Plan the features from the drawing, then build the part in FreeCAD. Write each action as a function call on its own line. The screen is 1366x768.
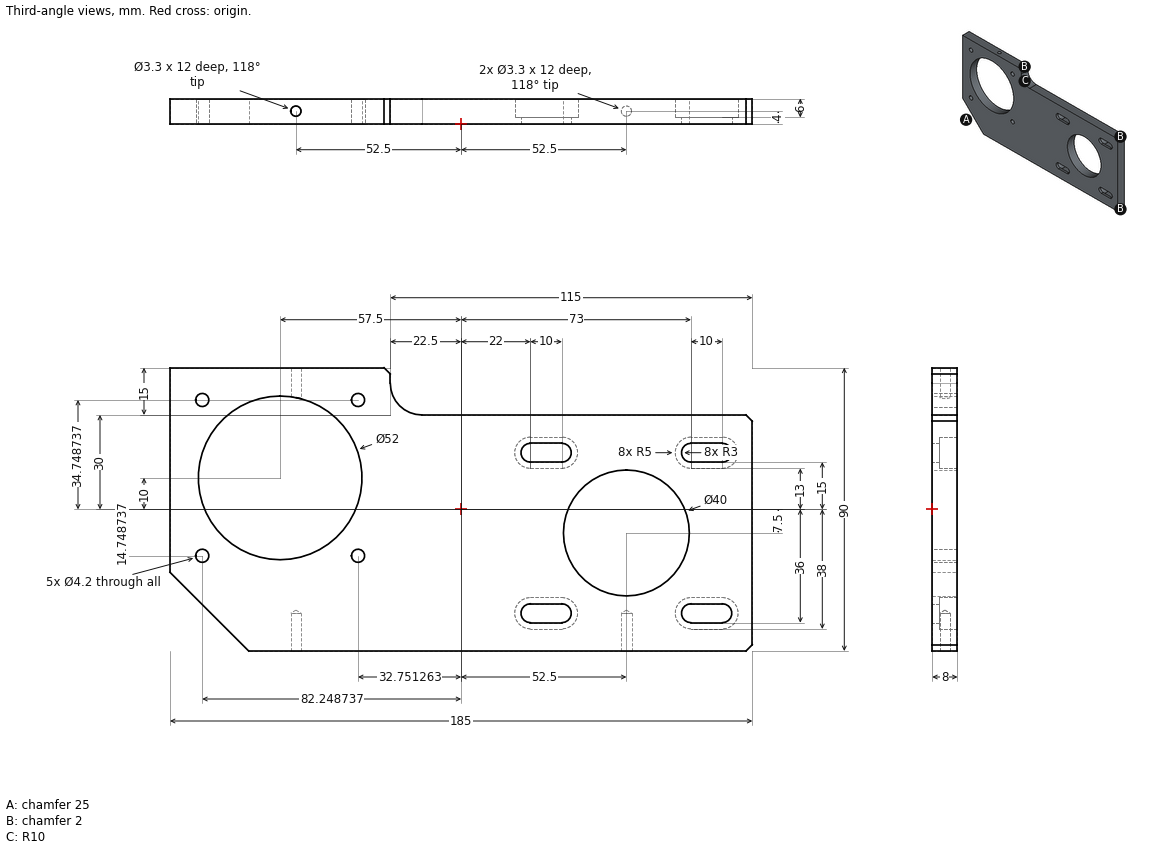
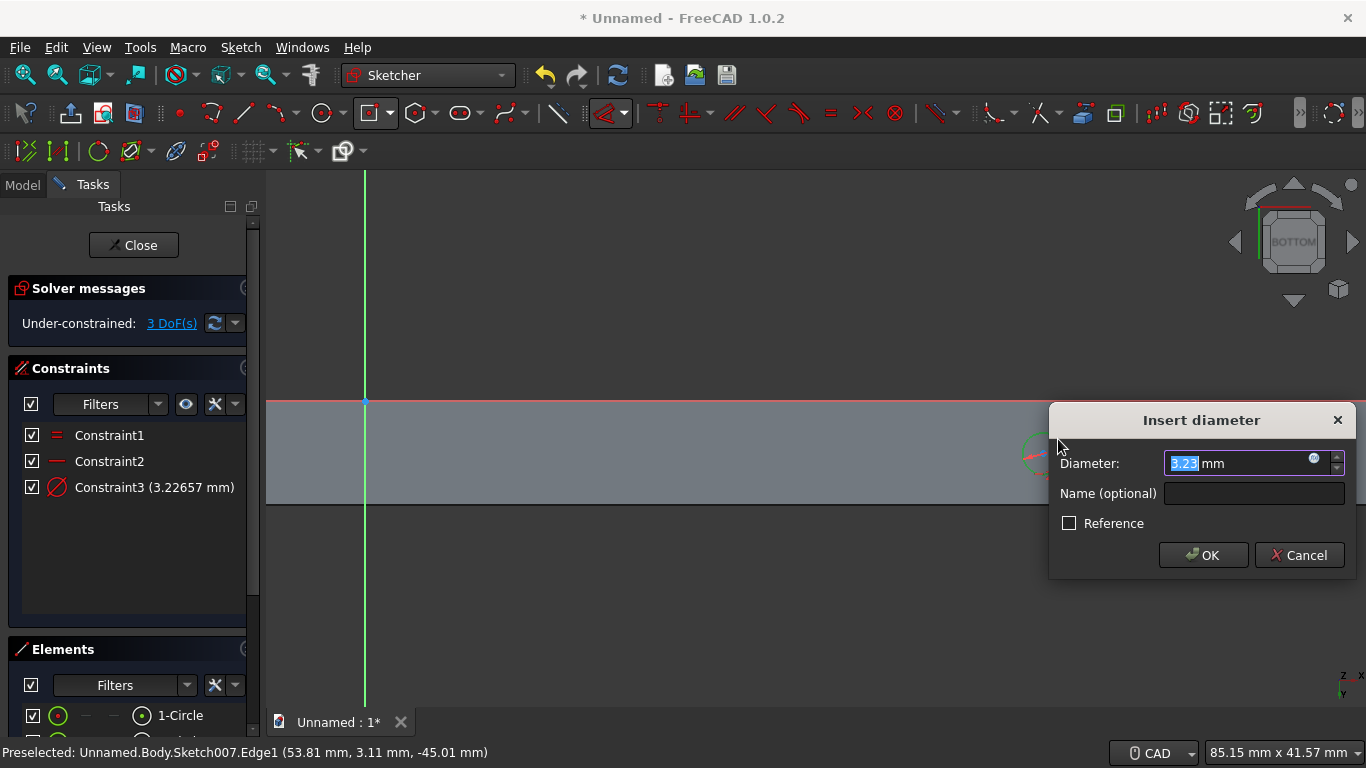
text(3.3)
key(Return)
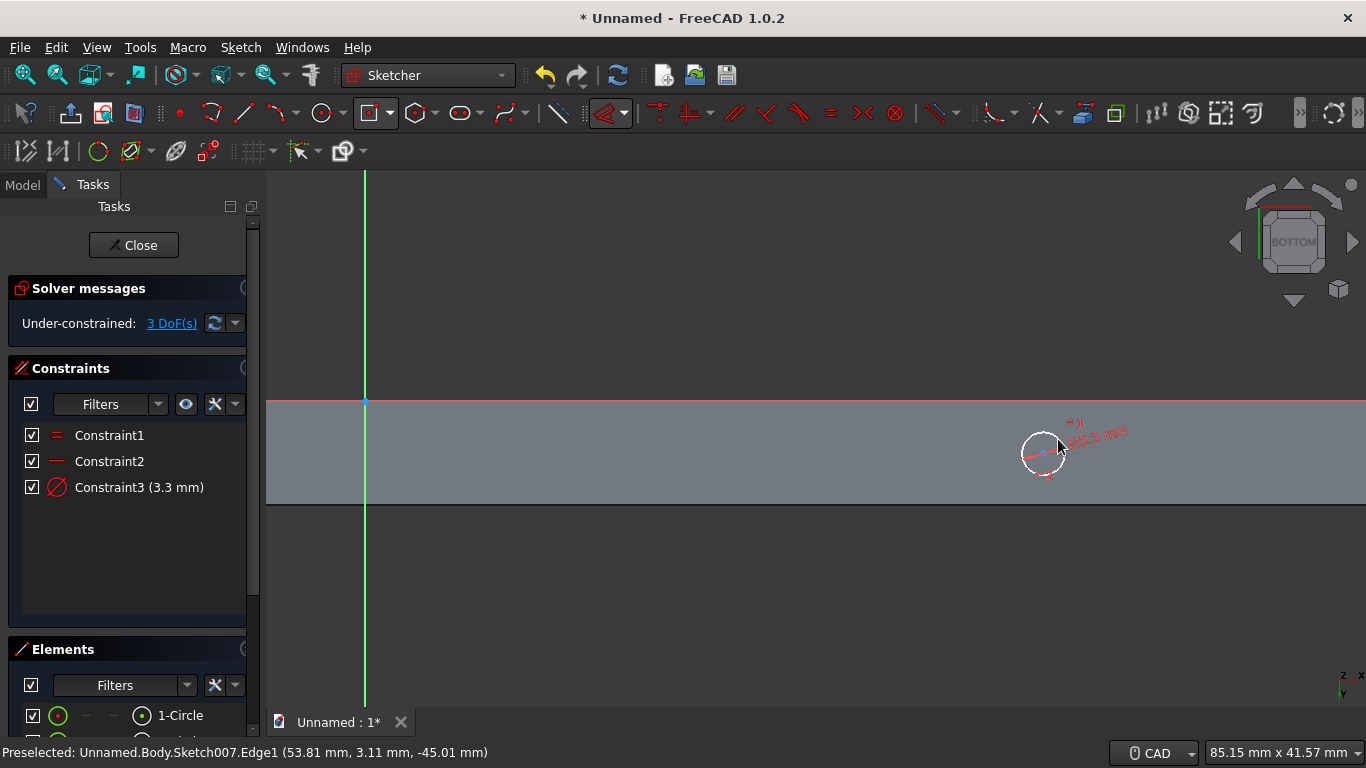
click(1043, 454)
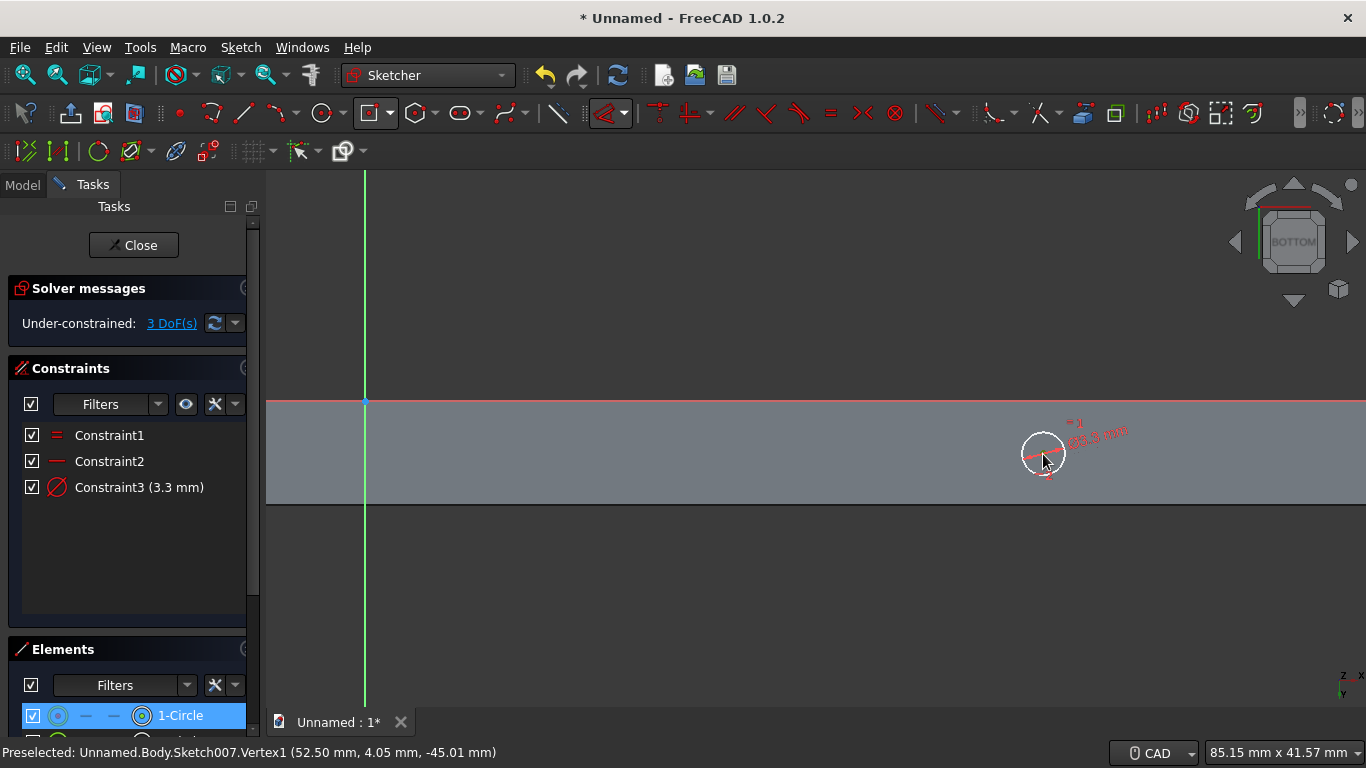
key(i)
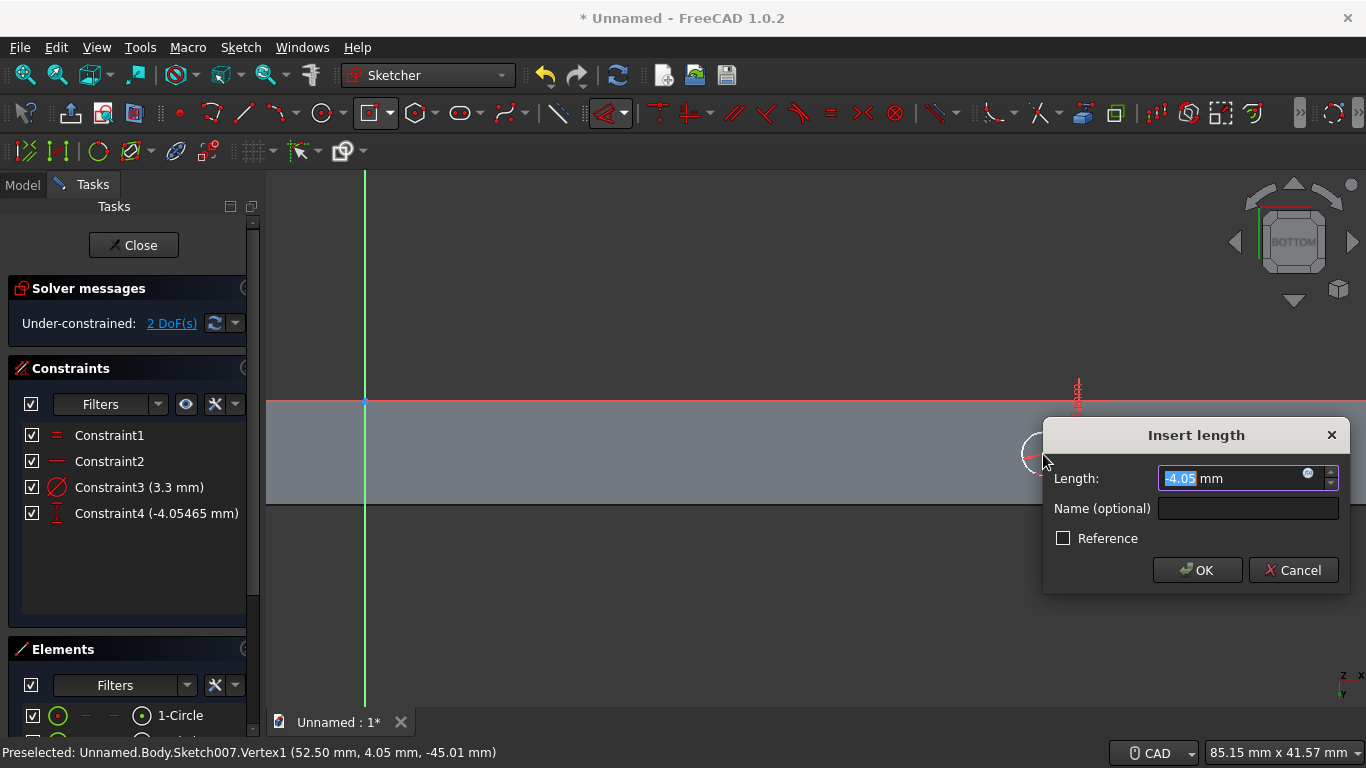
text(-4)
key(Return)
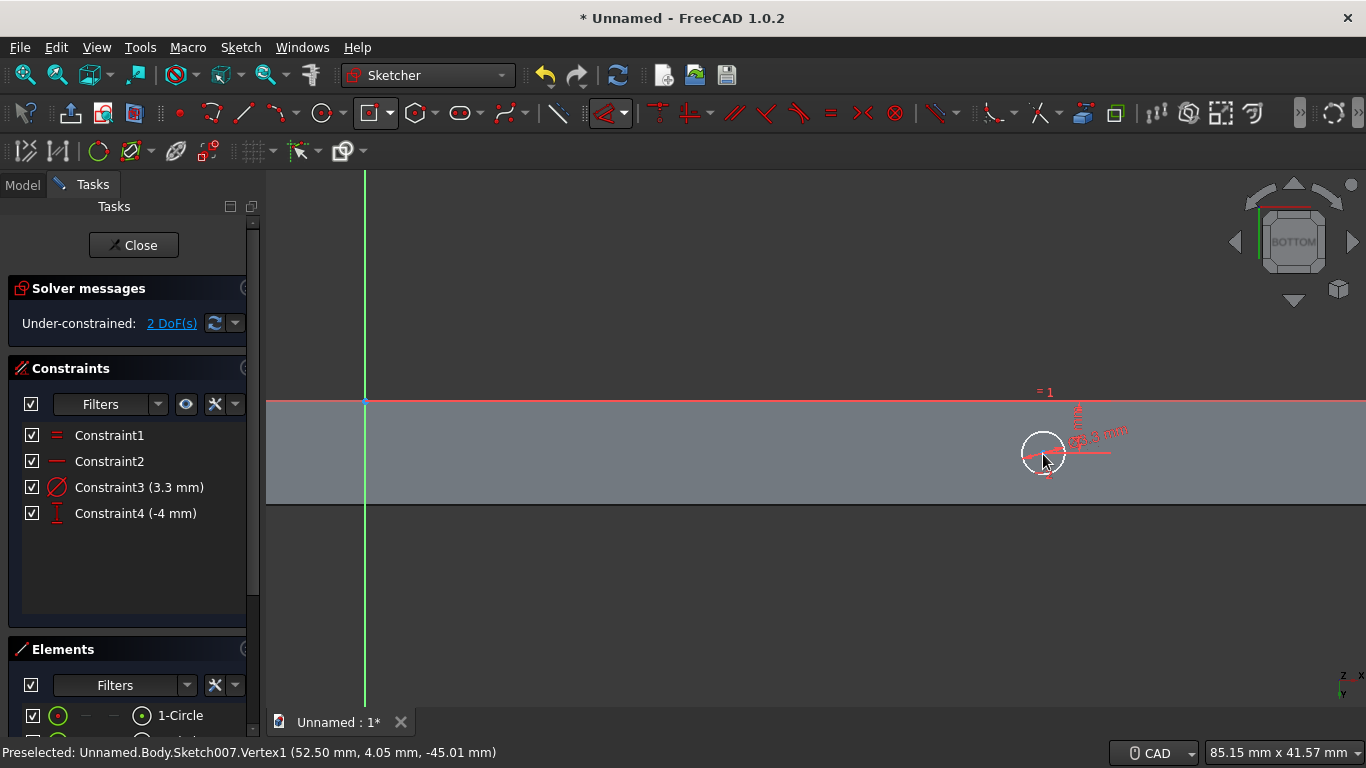
click(1043, 453)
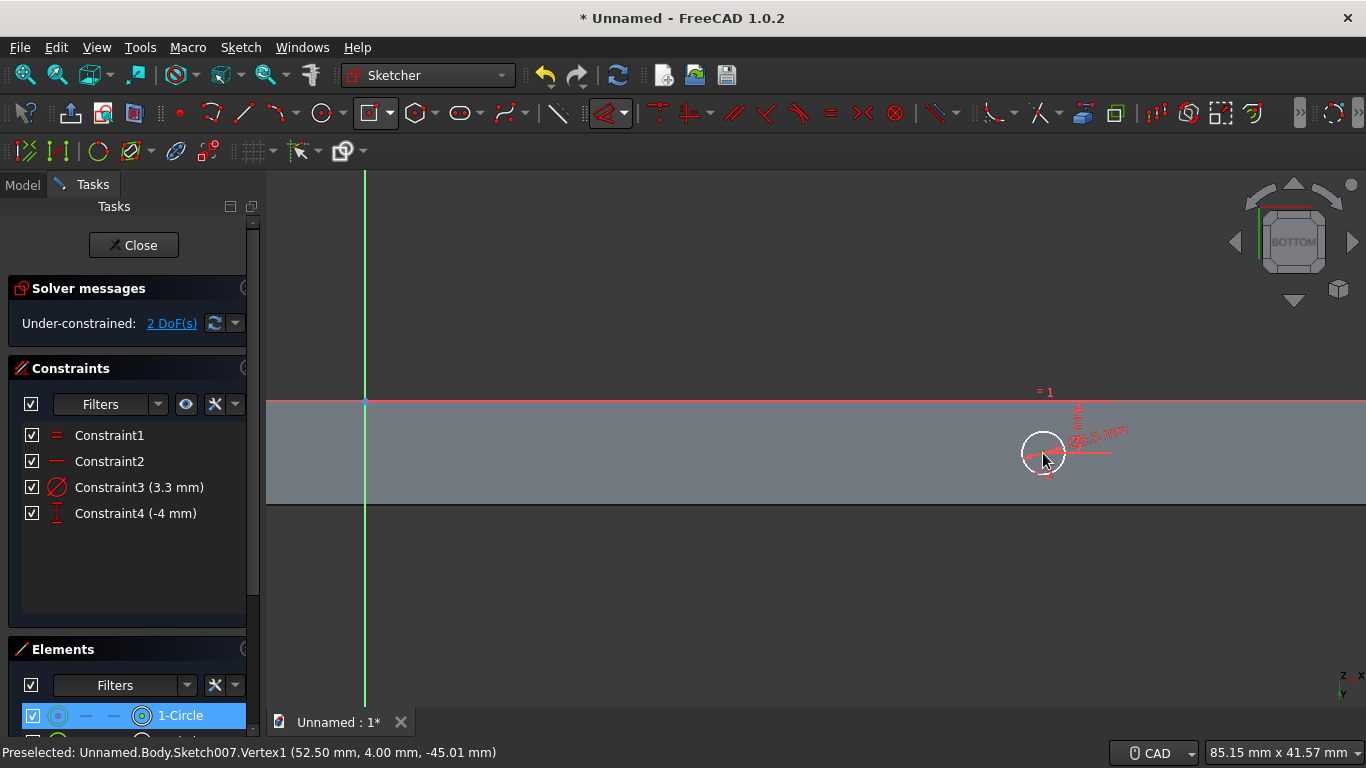
click(626, 114)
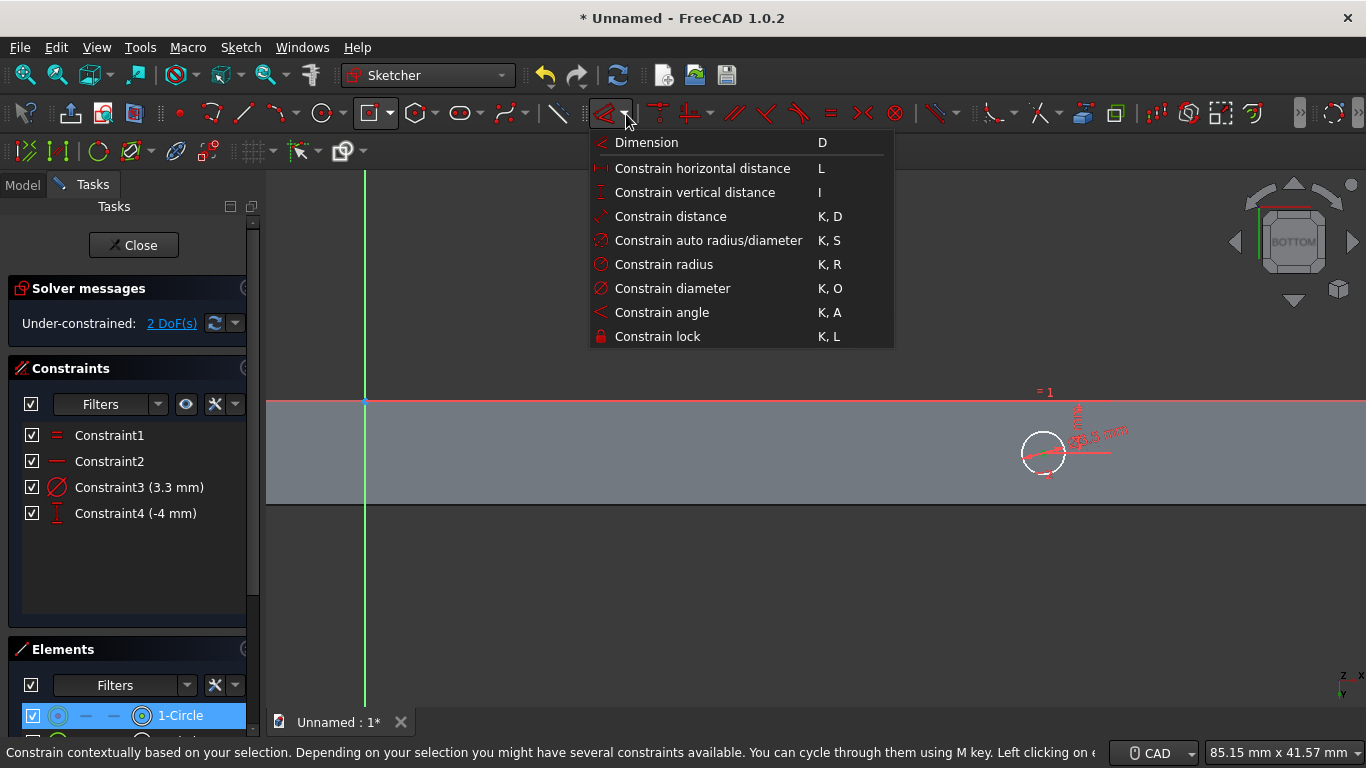
click(742, 168)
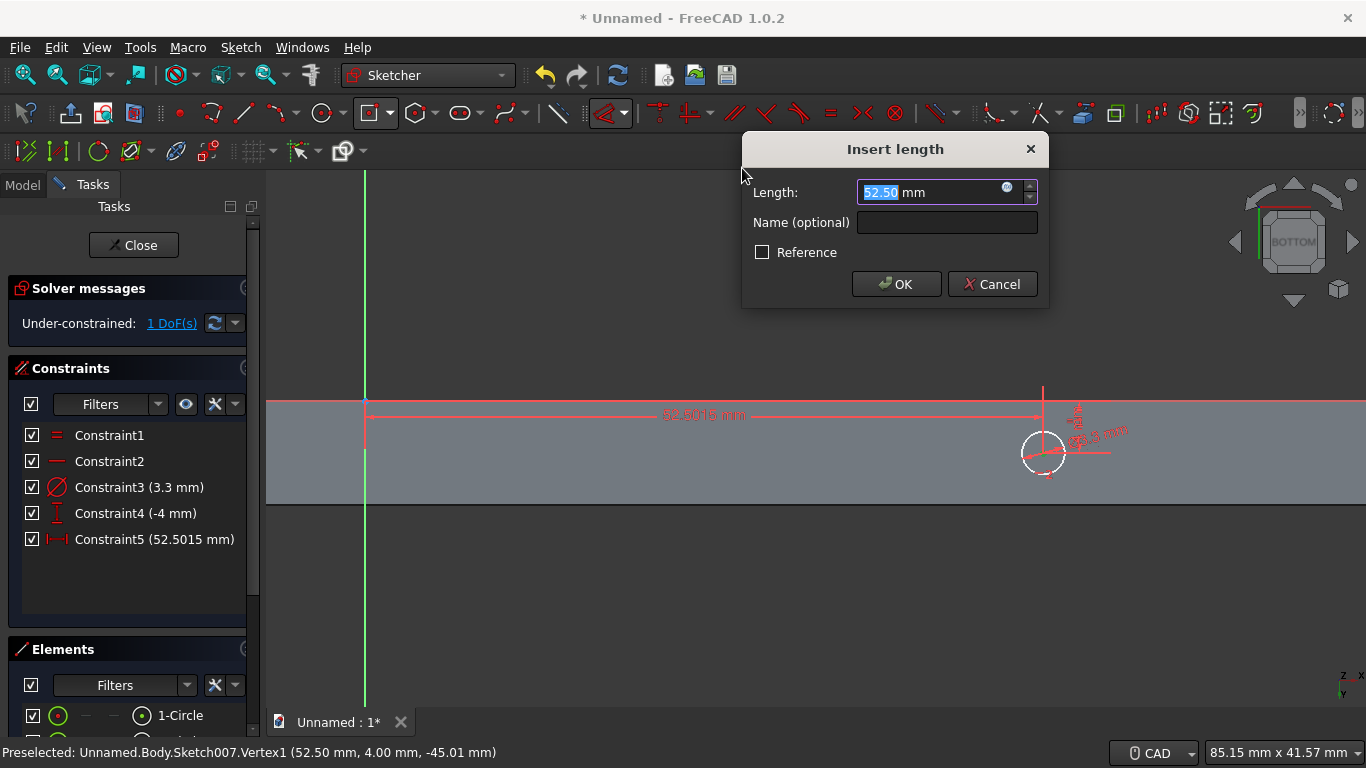
text(52.5)
key(Return)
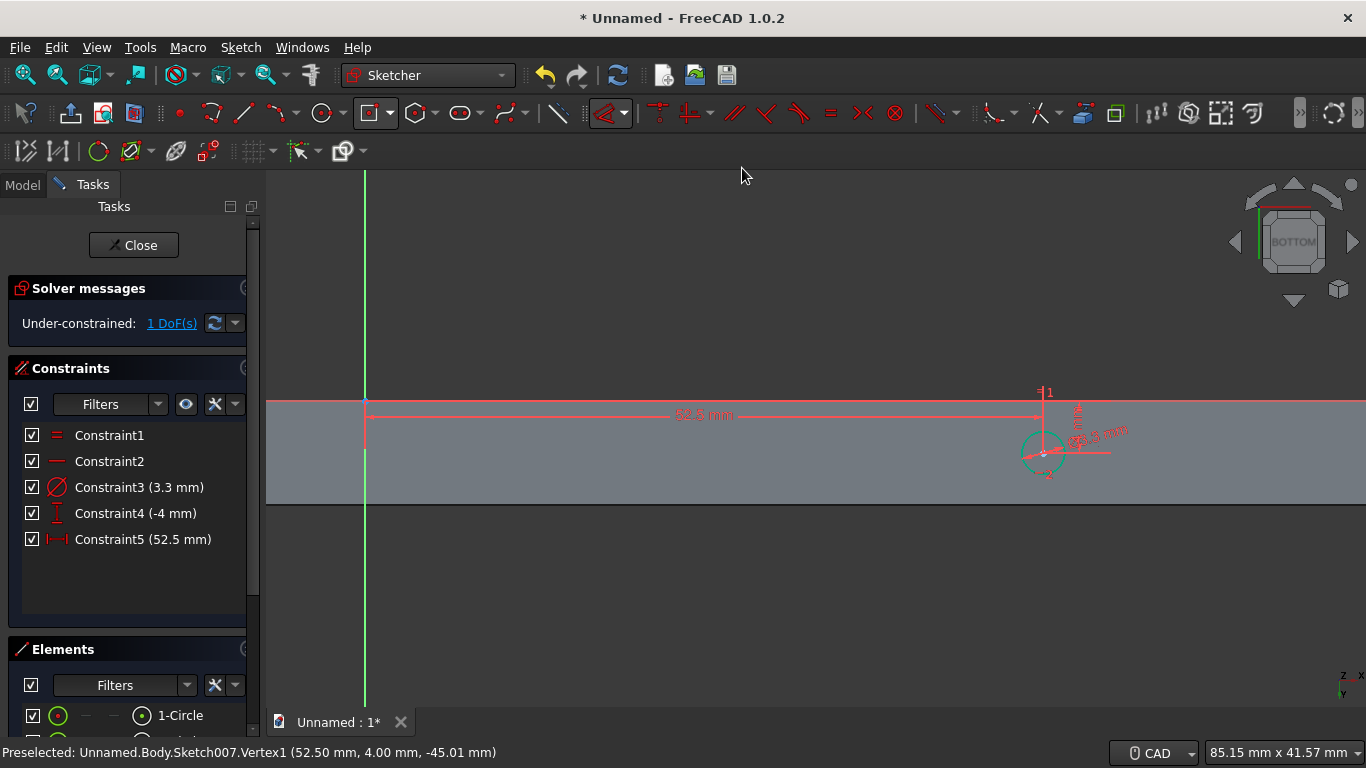
scroll(1059, 439, down, 4)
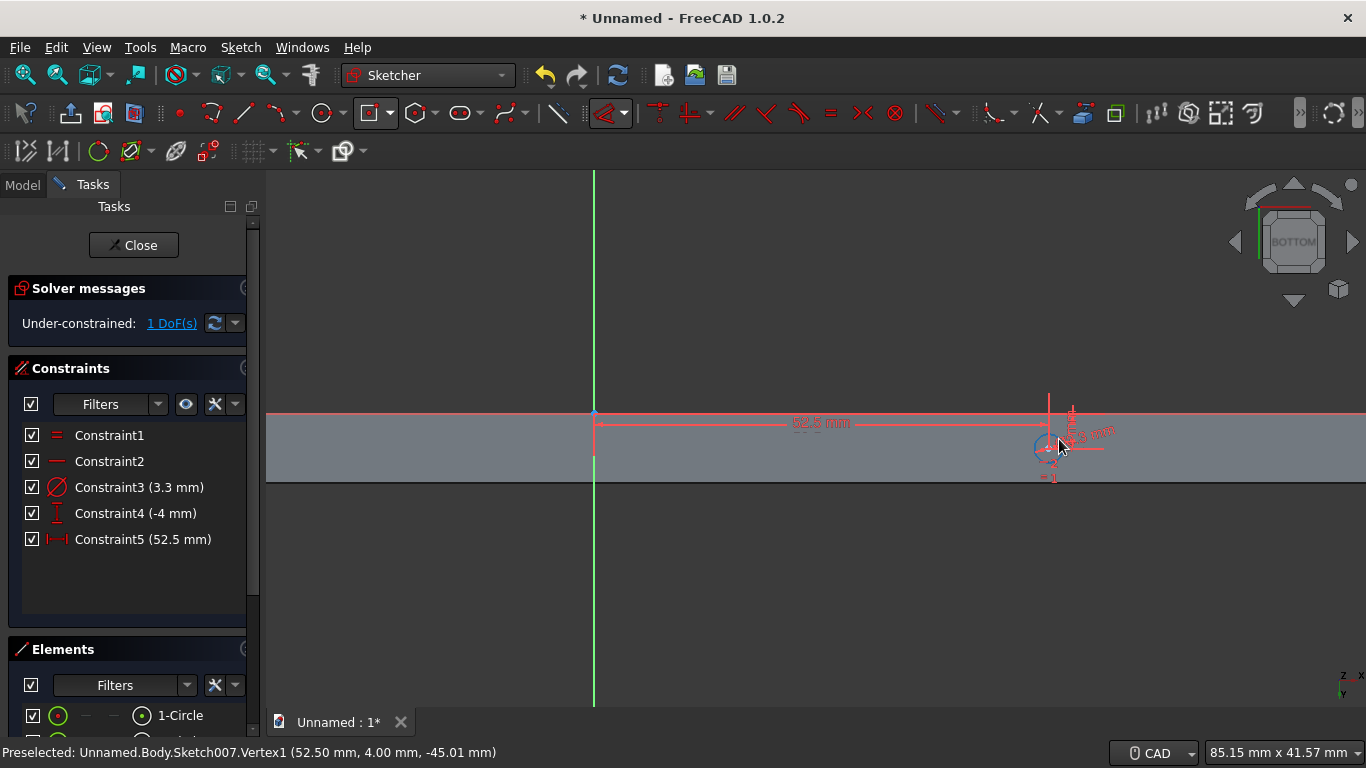
click(443, 446)